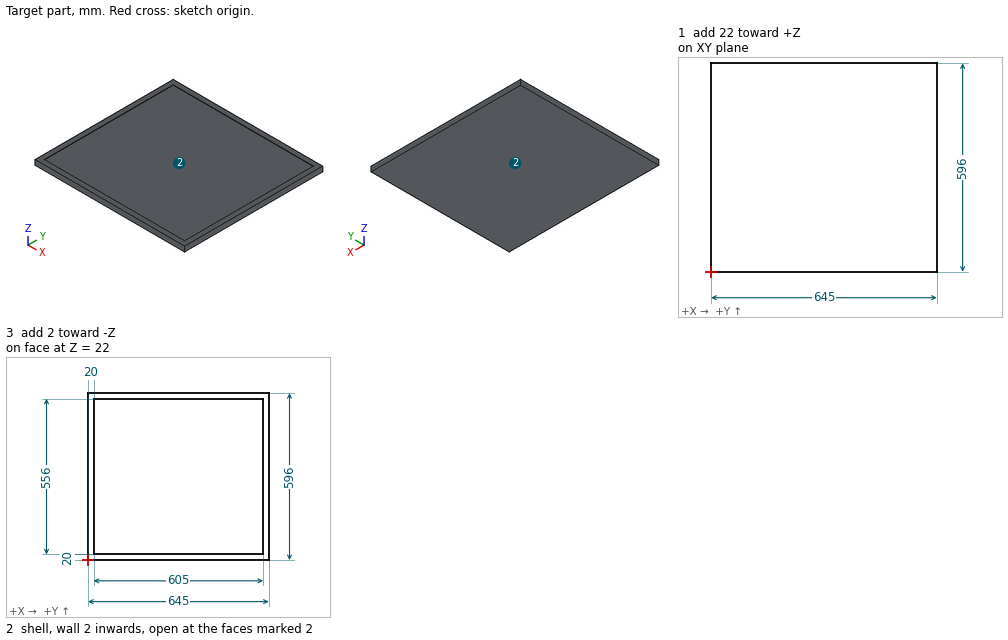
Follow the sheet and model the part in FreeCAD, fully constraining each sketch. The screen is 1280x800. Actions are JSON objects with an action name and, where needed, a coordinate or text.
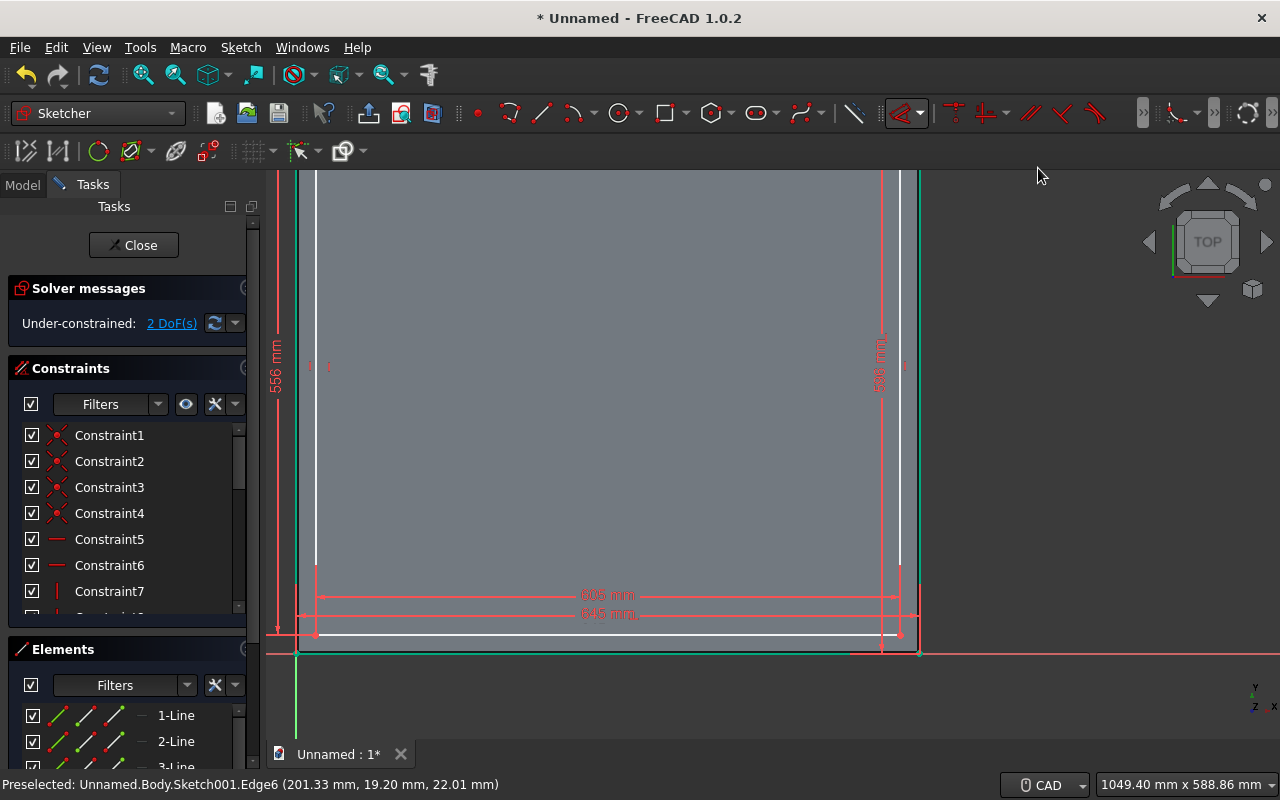
{"action": "scroll", "coordinate": [901, 635], "scroll_direction": "down", "scroll_amount": 2}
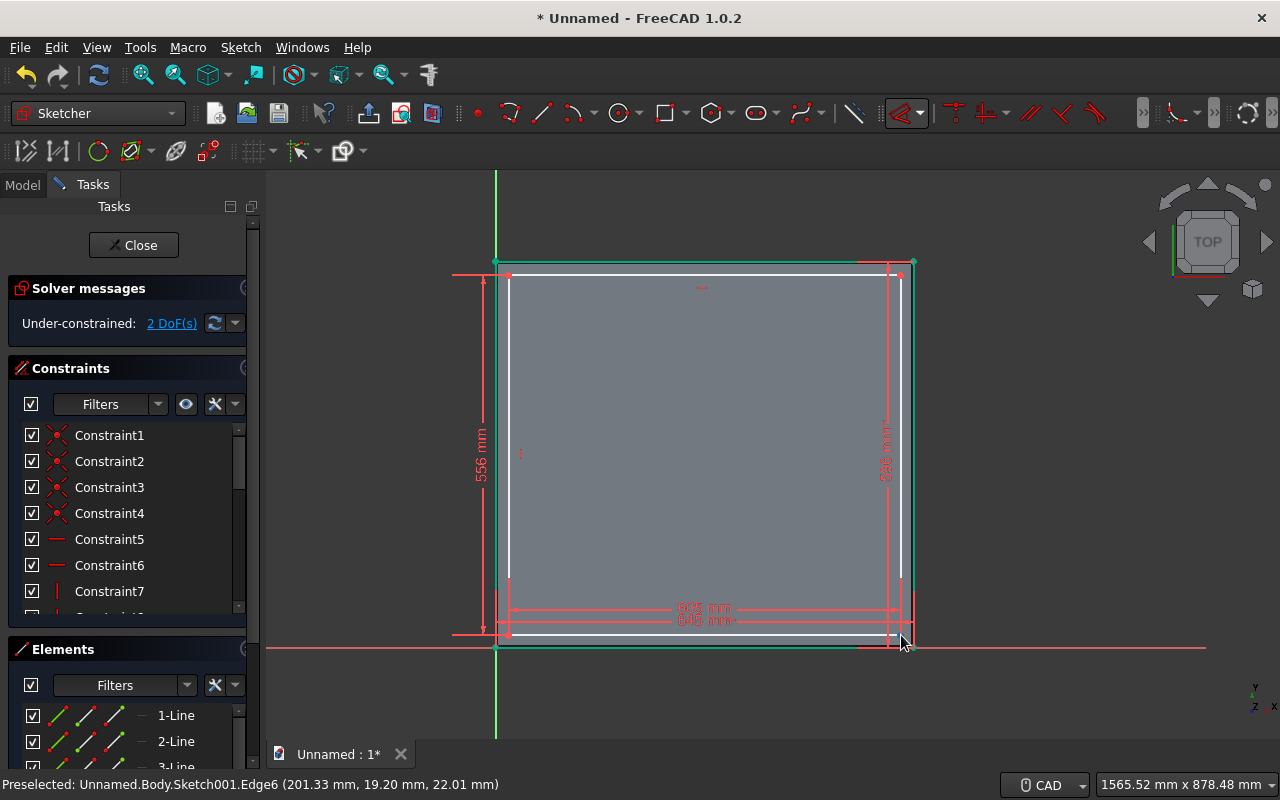
{"action": "scroll", "coordinate": [509, 275], "scroll_direction": "up", "scroll_amount": 6}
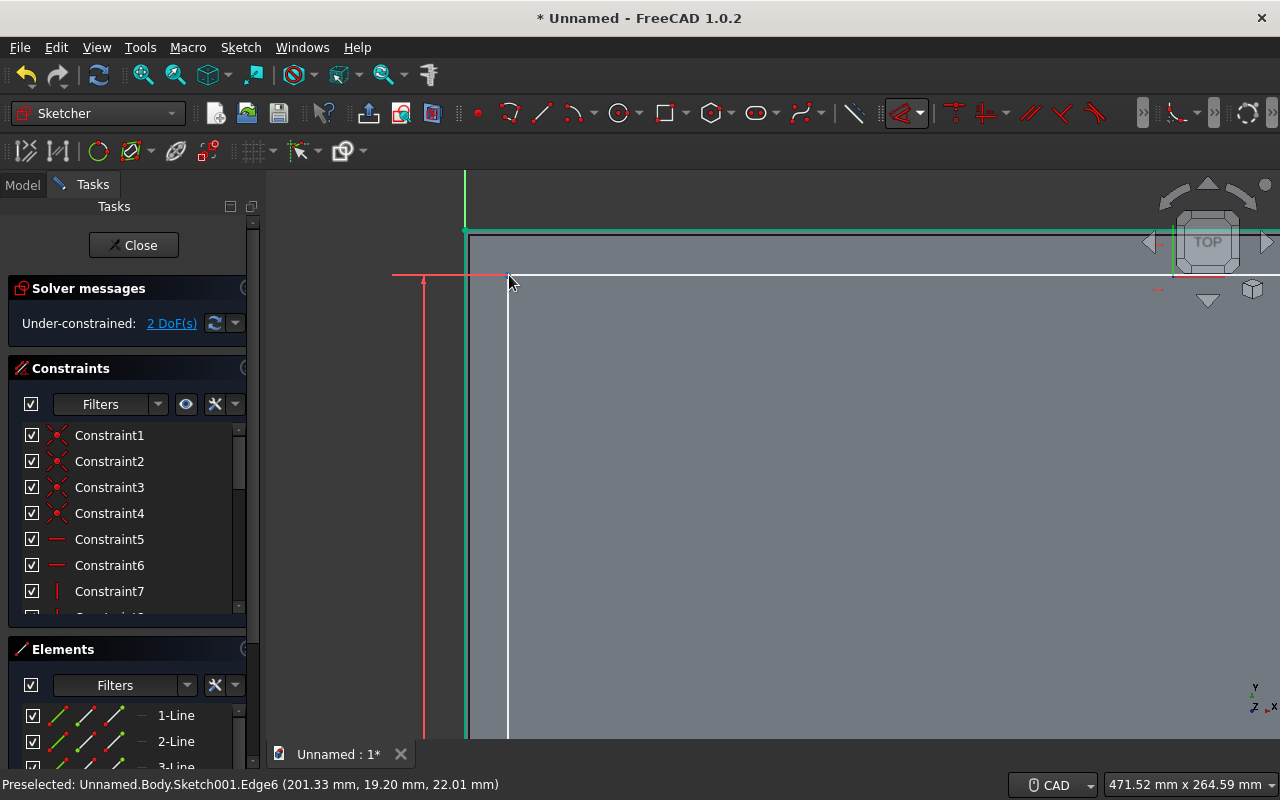
{"action": "left_click", "coordinate": [508, 275]}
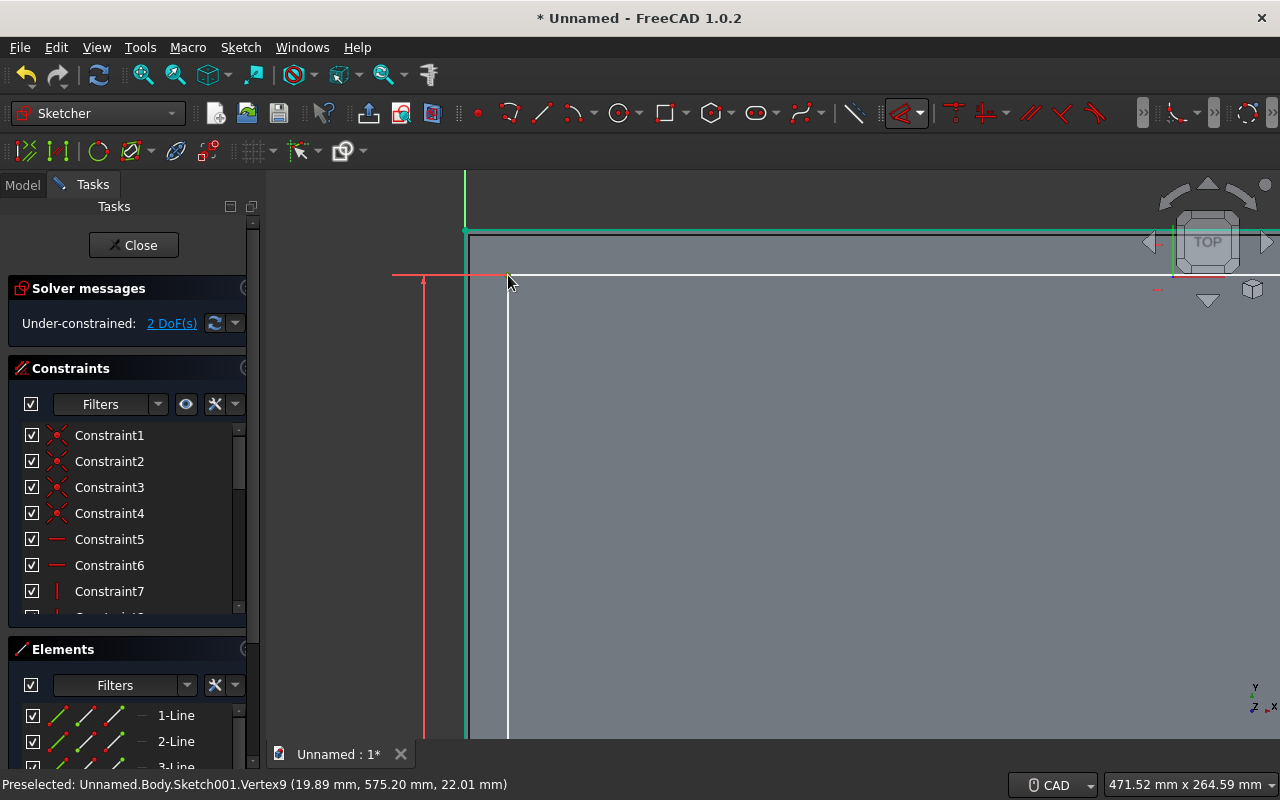
{"action": "left_click", "coordinate": [922, 114]}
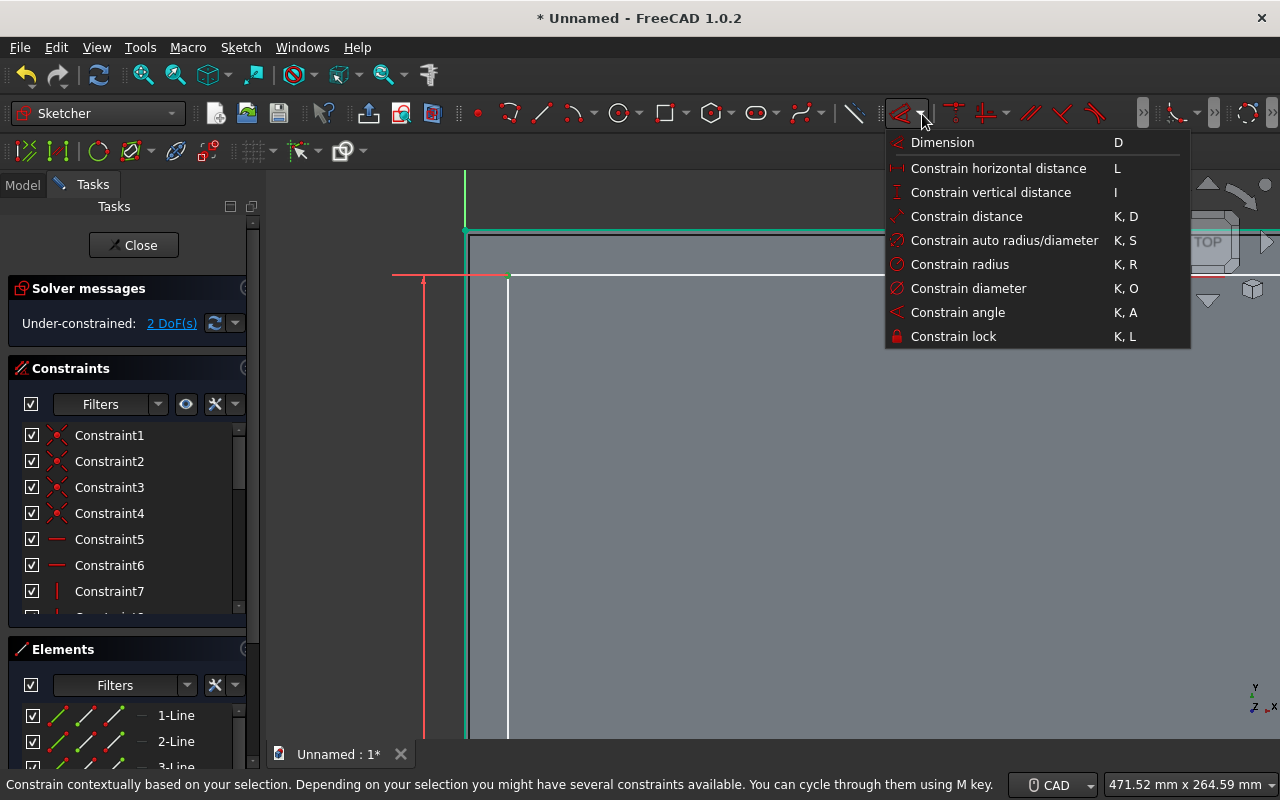
{"action": "left_click", "coordinate": [1038, 168]}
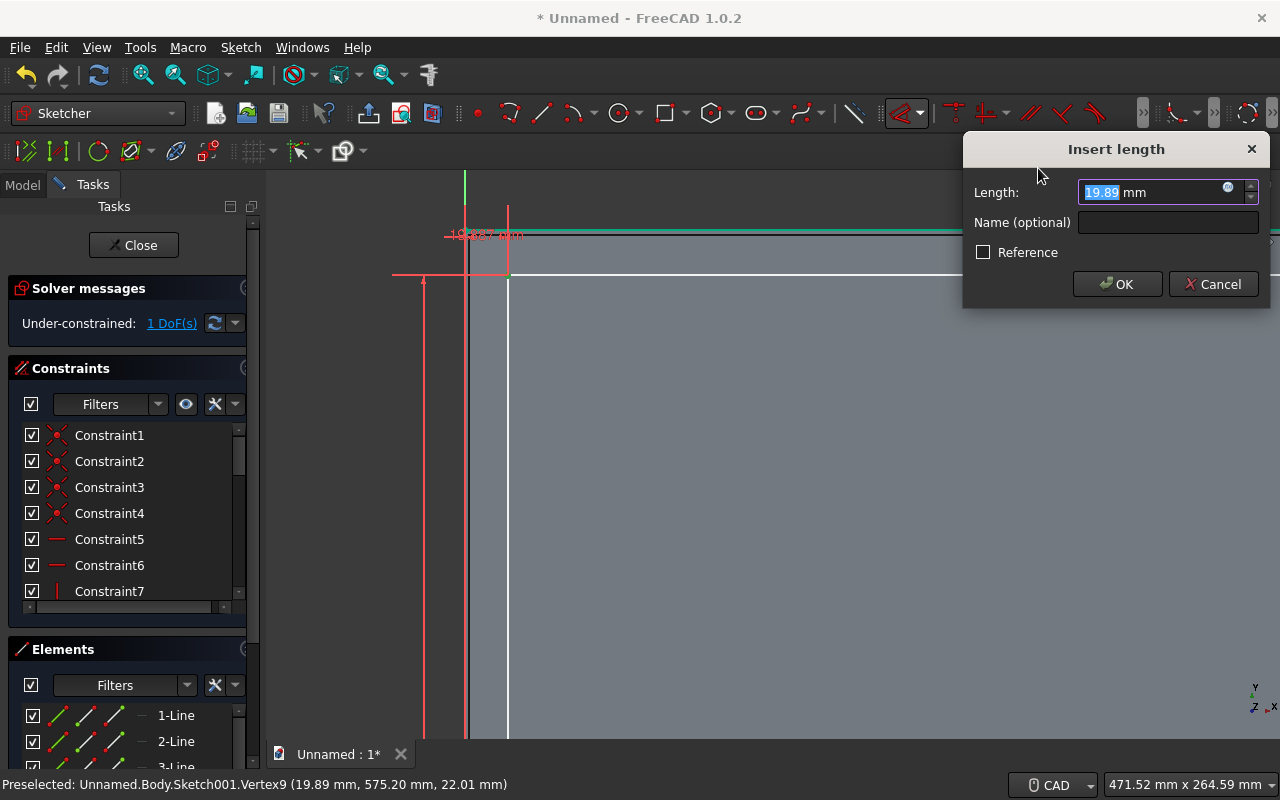
{"action": "type", "text": "20"}
{"action": "key", "text": "Return"}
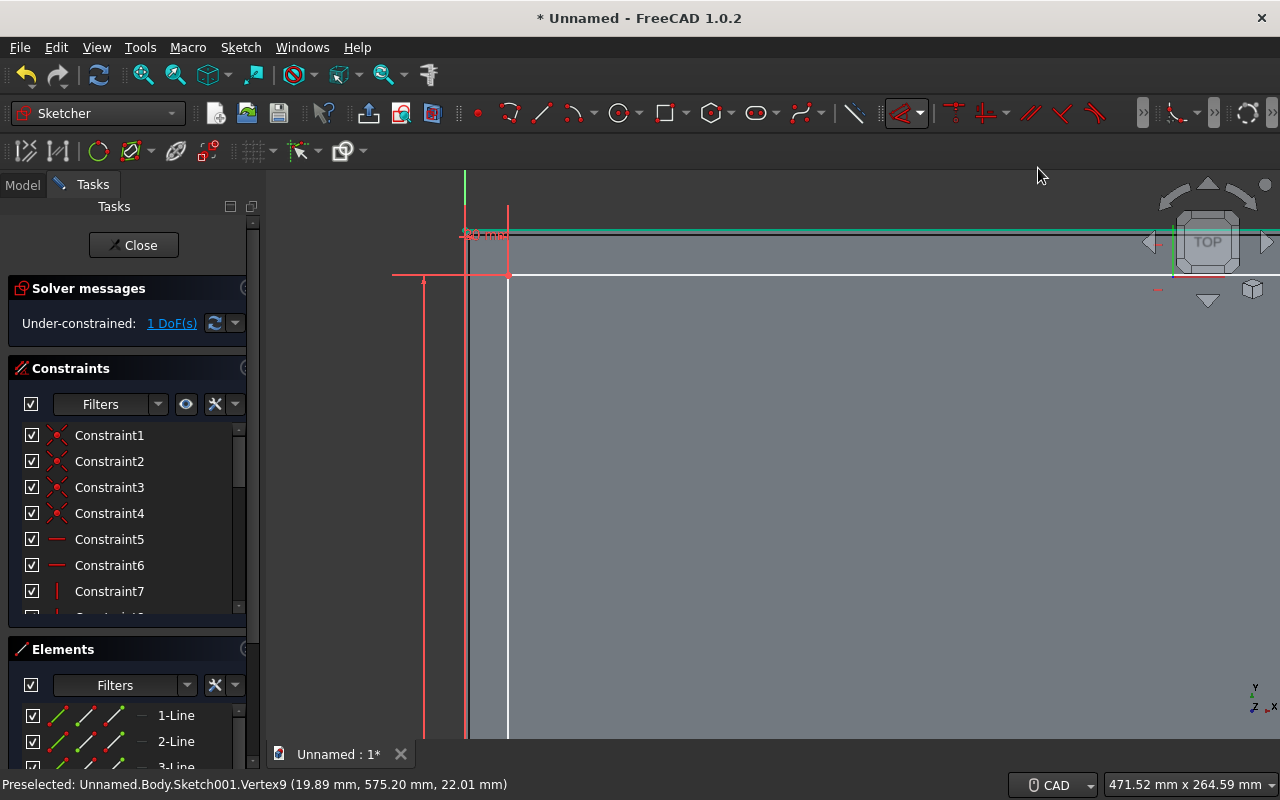
{"action": "scroll", "coordinate": [509, 275], "scroll_direction": "down", "scroll_amount": 6}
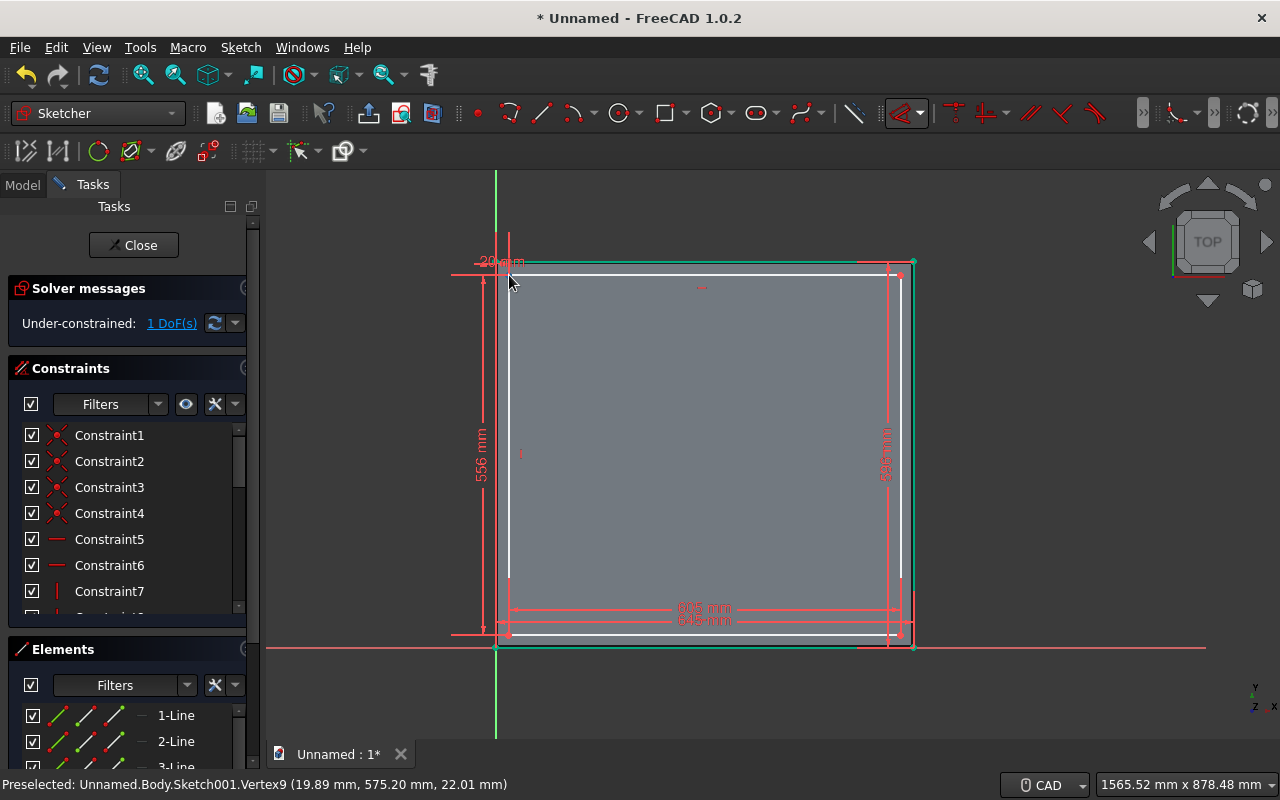
{"action": "scroll", "coordinate": [509, 635], "scroll_direction": "up", "scroll_amount": 6}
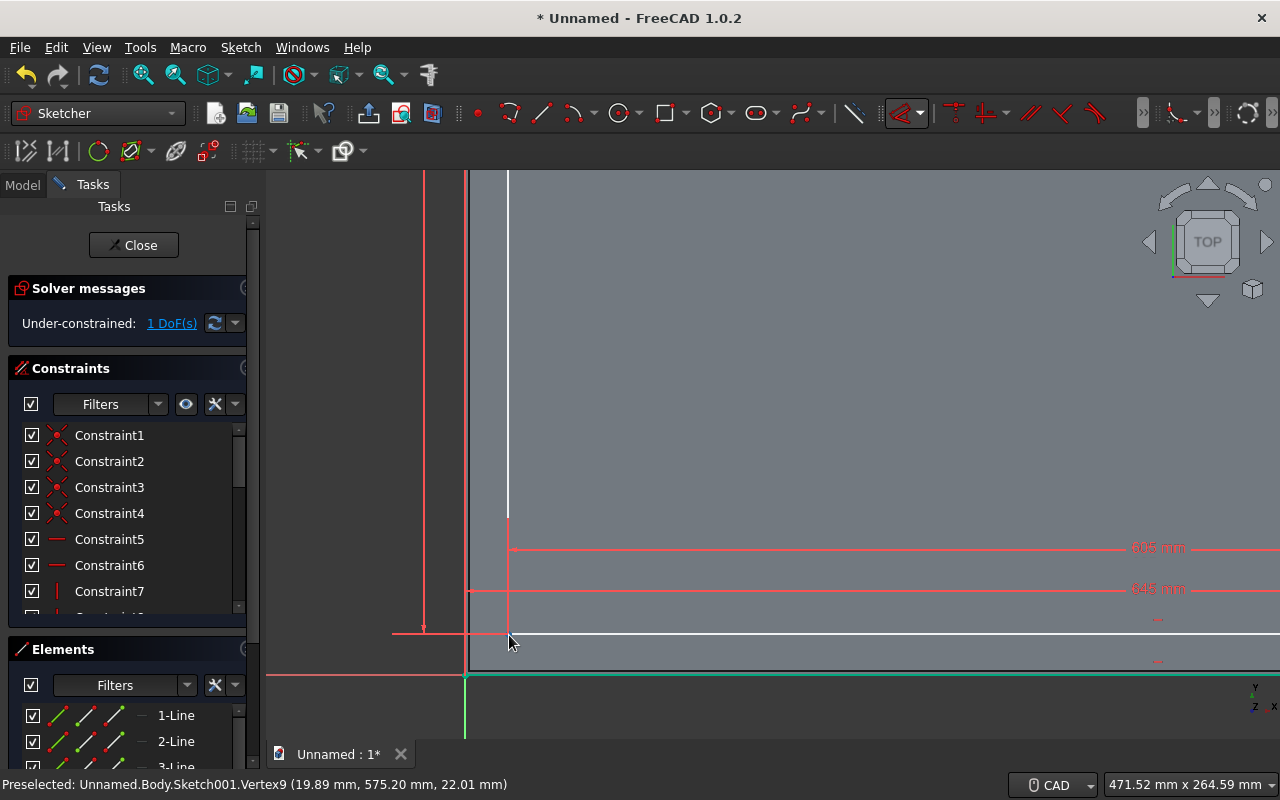
{"action": "left_click", "coordinate": [508, 634]}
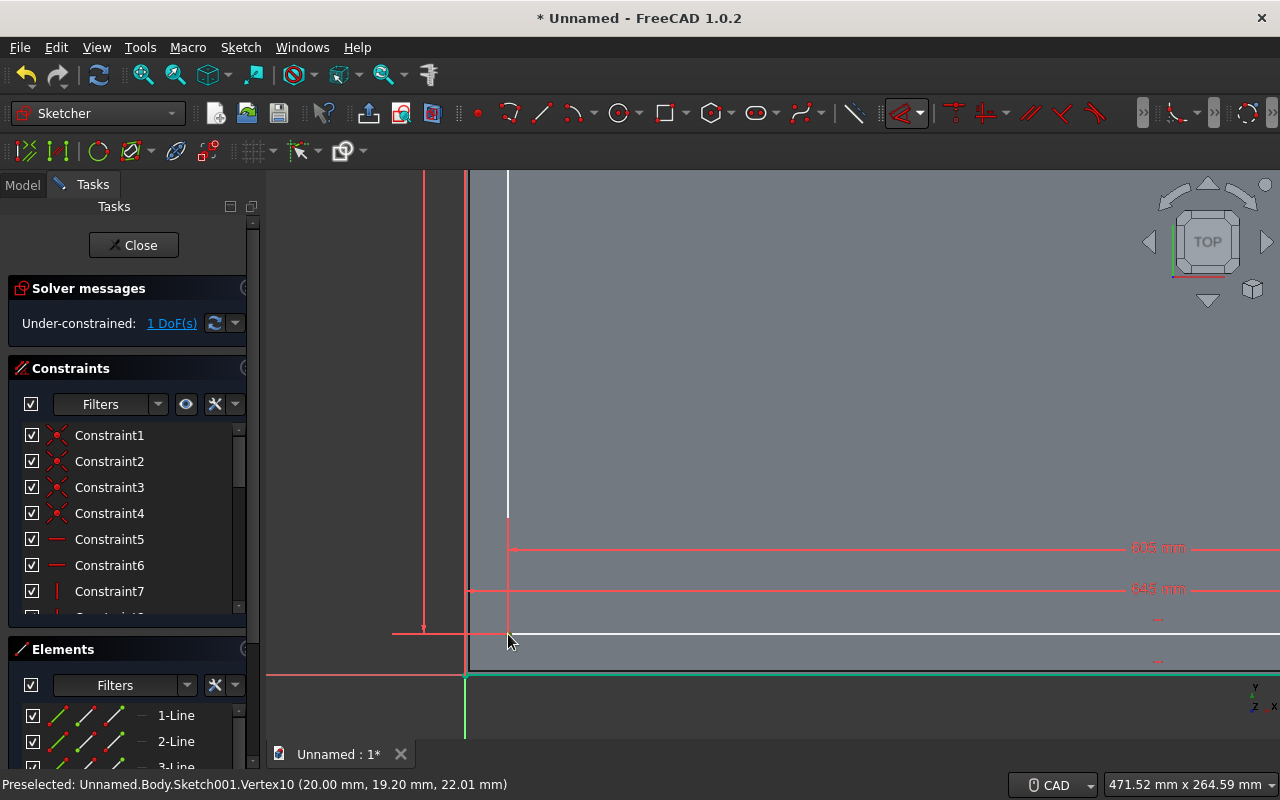
{"action": "key", "text": "i"}